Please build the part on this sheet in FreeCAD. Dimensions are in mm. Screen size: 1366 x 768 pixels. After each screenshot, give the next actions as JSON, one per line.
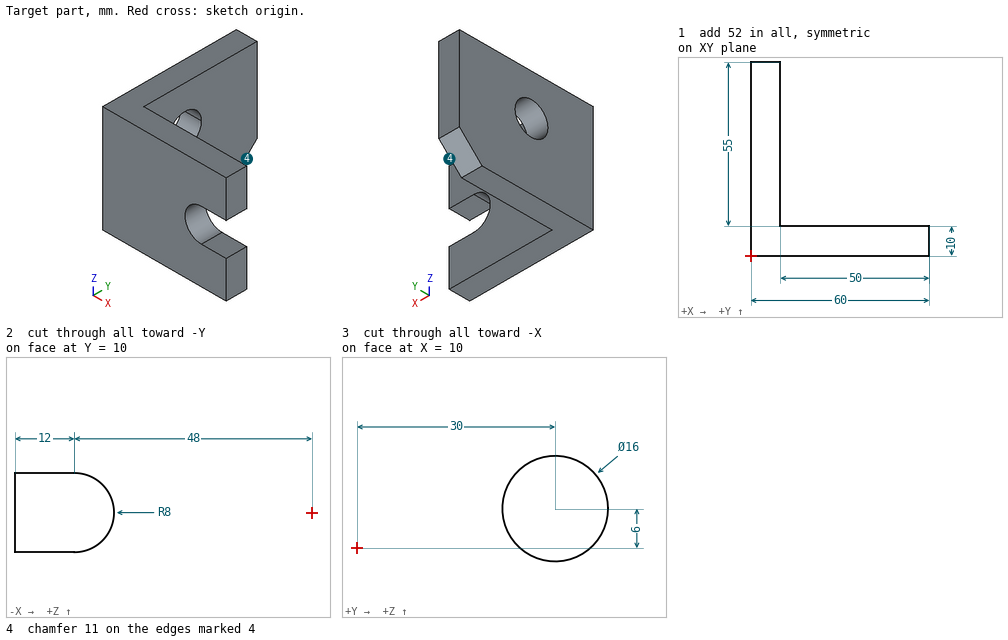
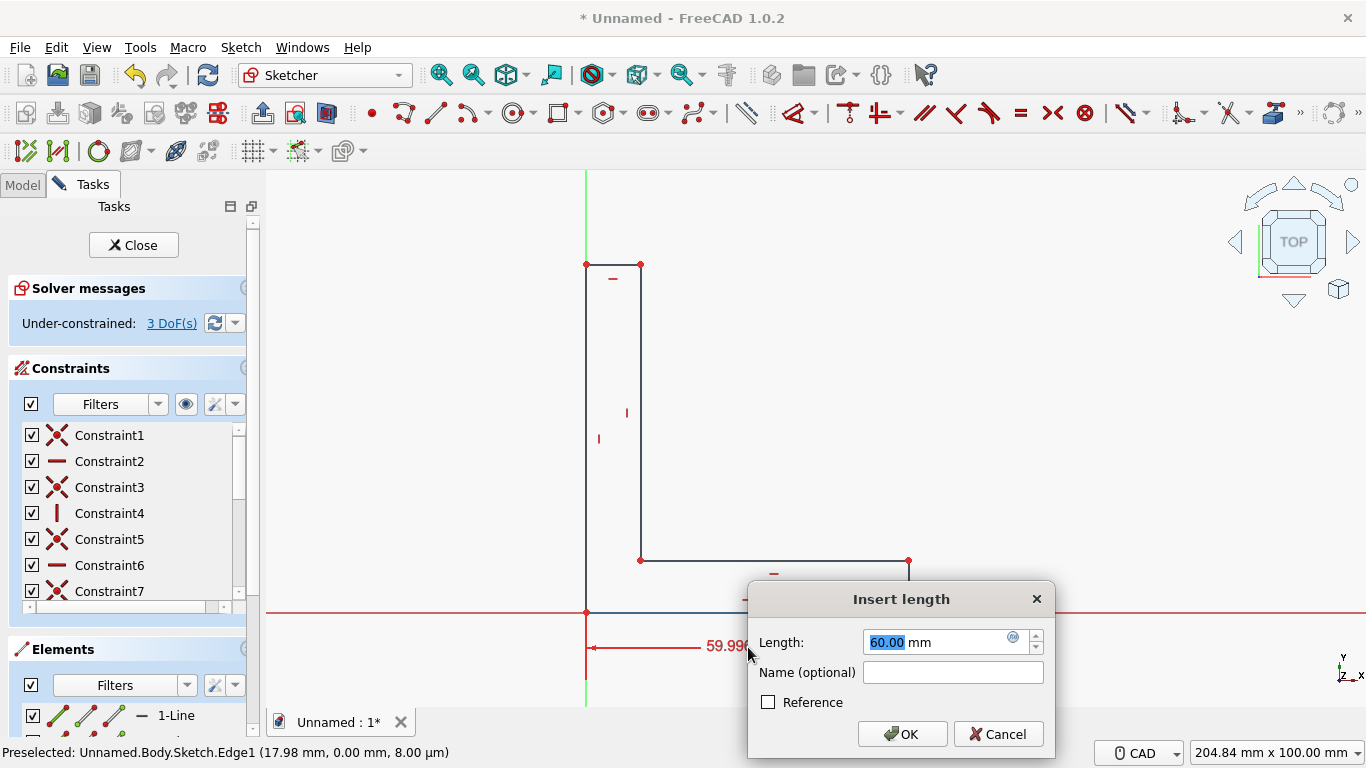
{"action": "type", "text": "60"}
{"action": "key", "text": "Return"}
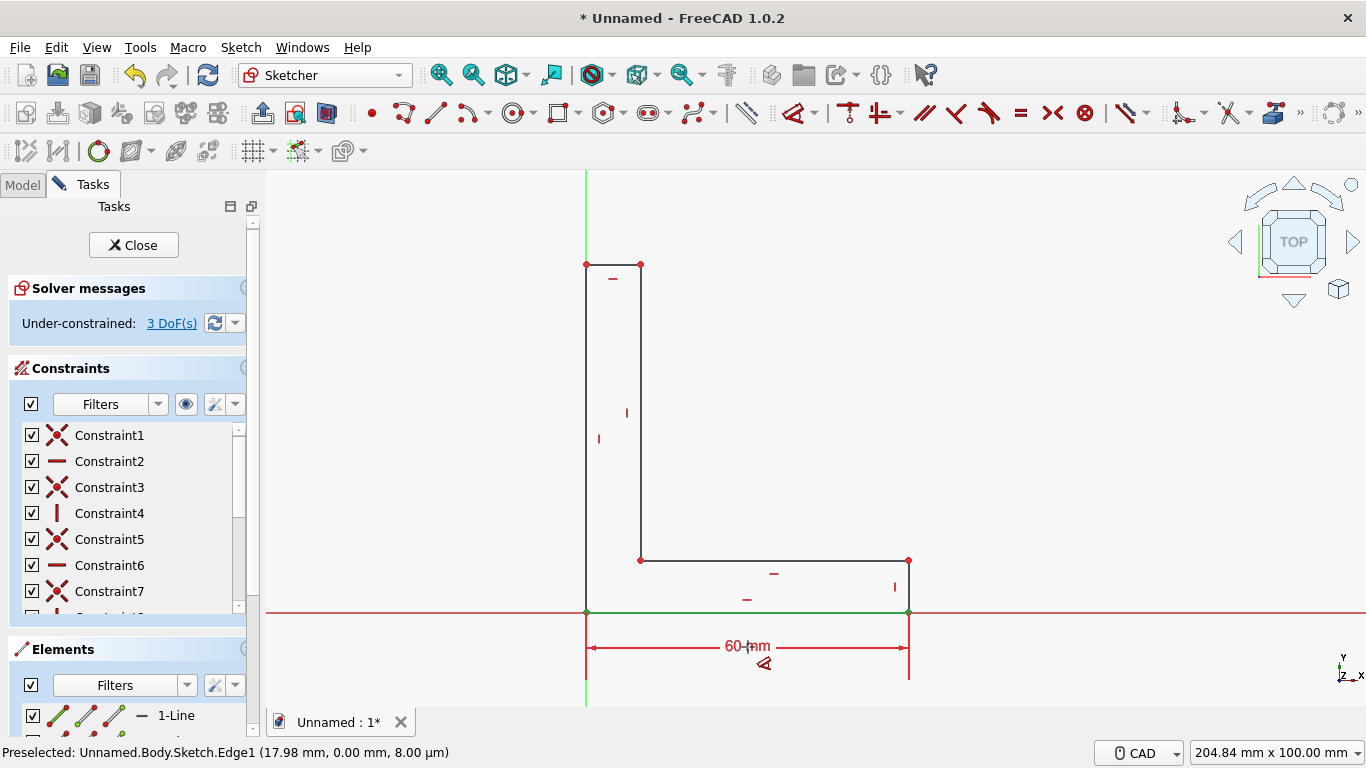
{"action": "left_click", "coordinate": [909, 597]}
{"action": "left_click", "coordinate": [943, 587]}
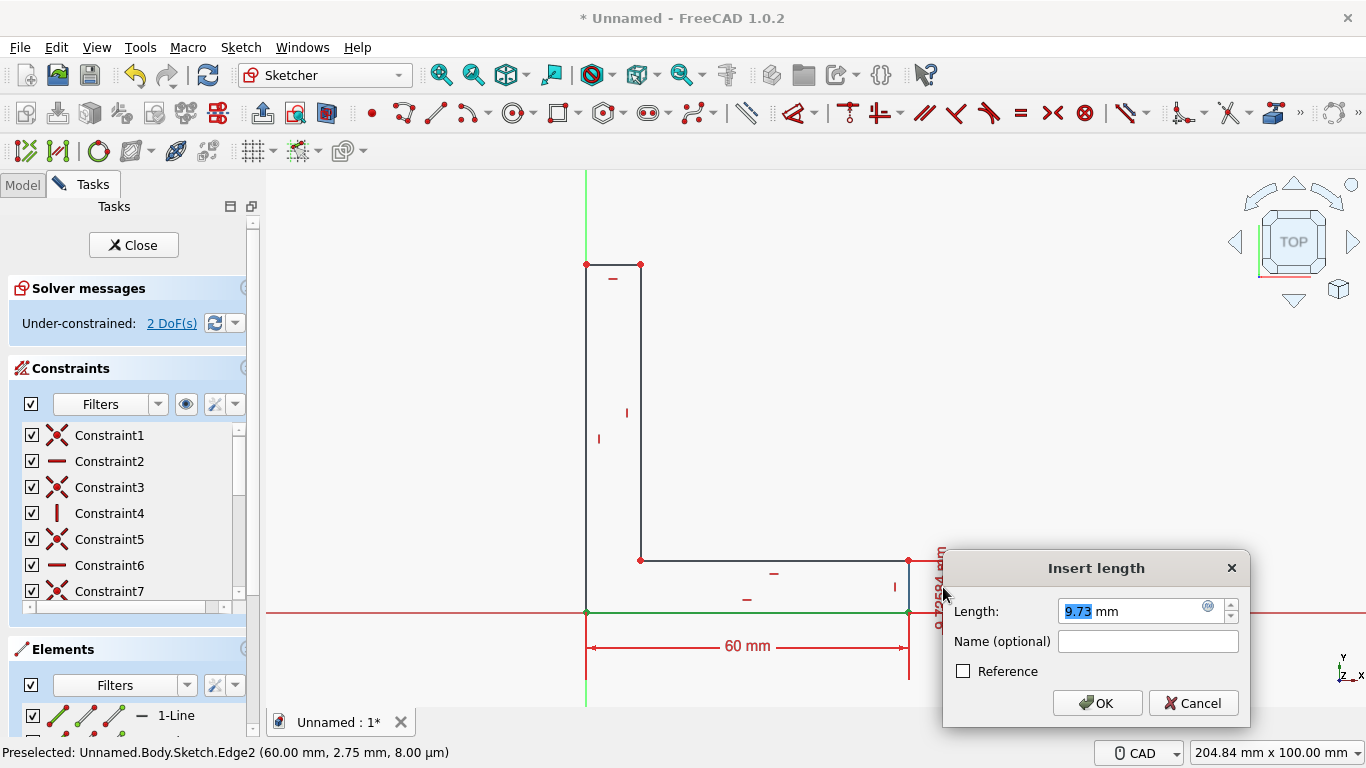
{"action": "type", "text": "10"}
{"action": "key", "text": "Return"}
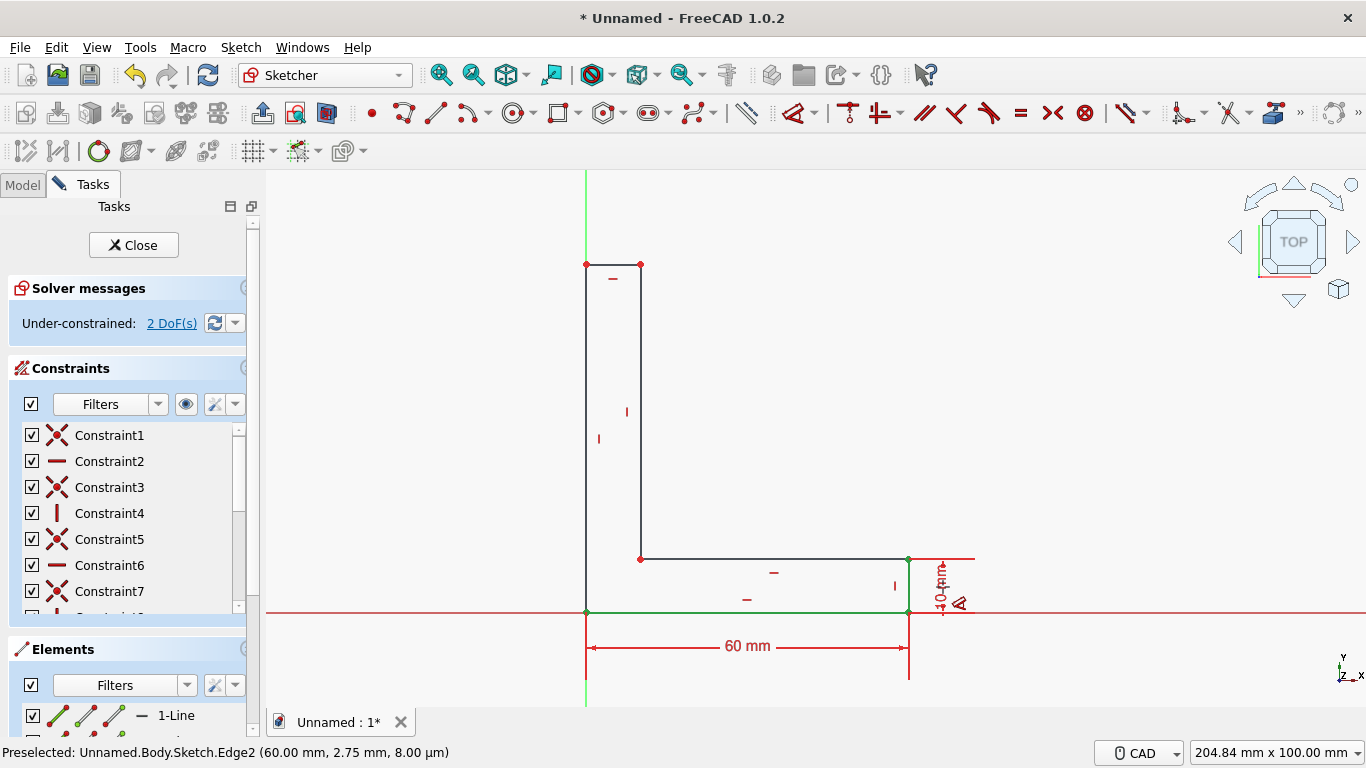
{"action": "left_click", "coordinate": [828, 559]}
{"action": "left_click", "coordinate": [775, 593]}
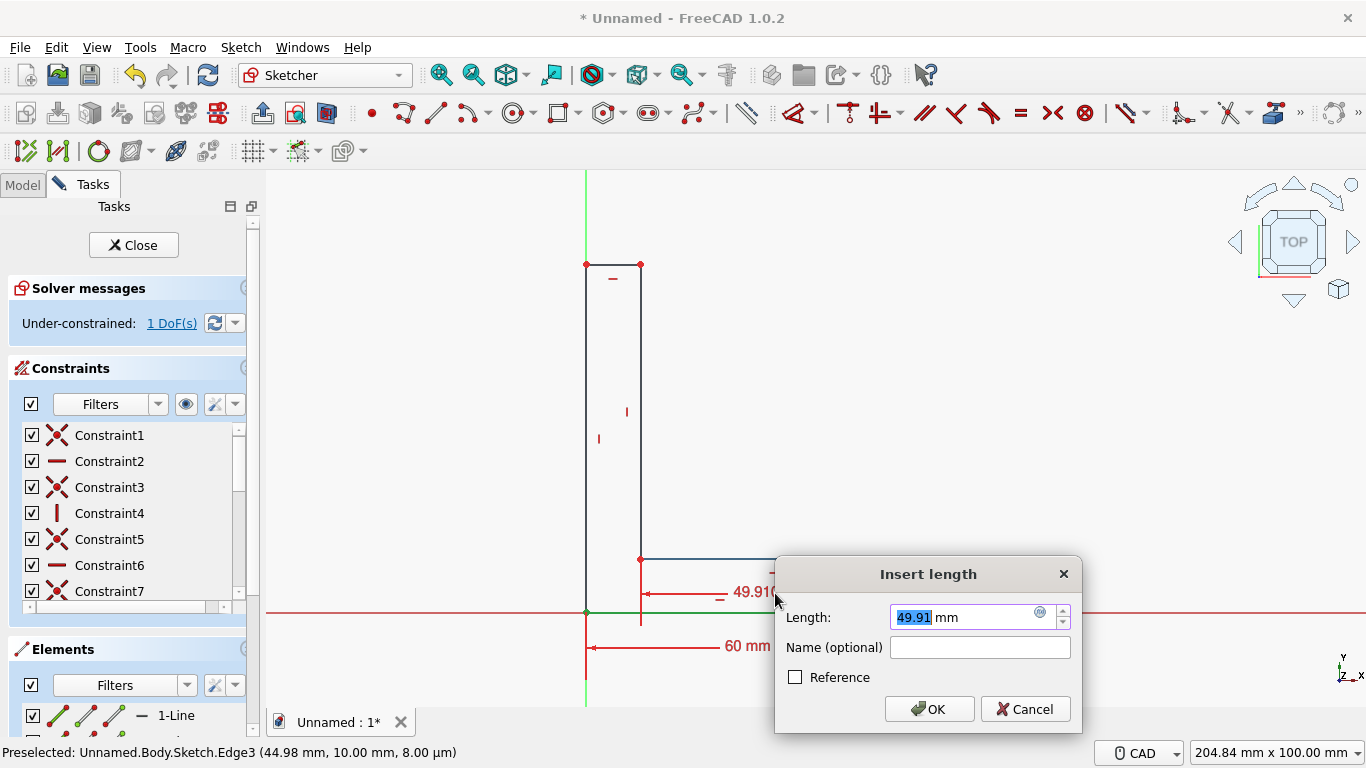
{"action": "type", "text": "50"}
{"action": "key", "text": "Return"}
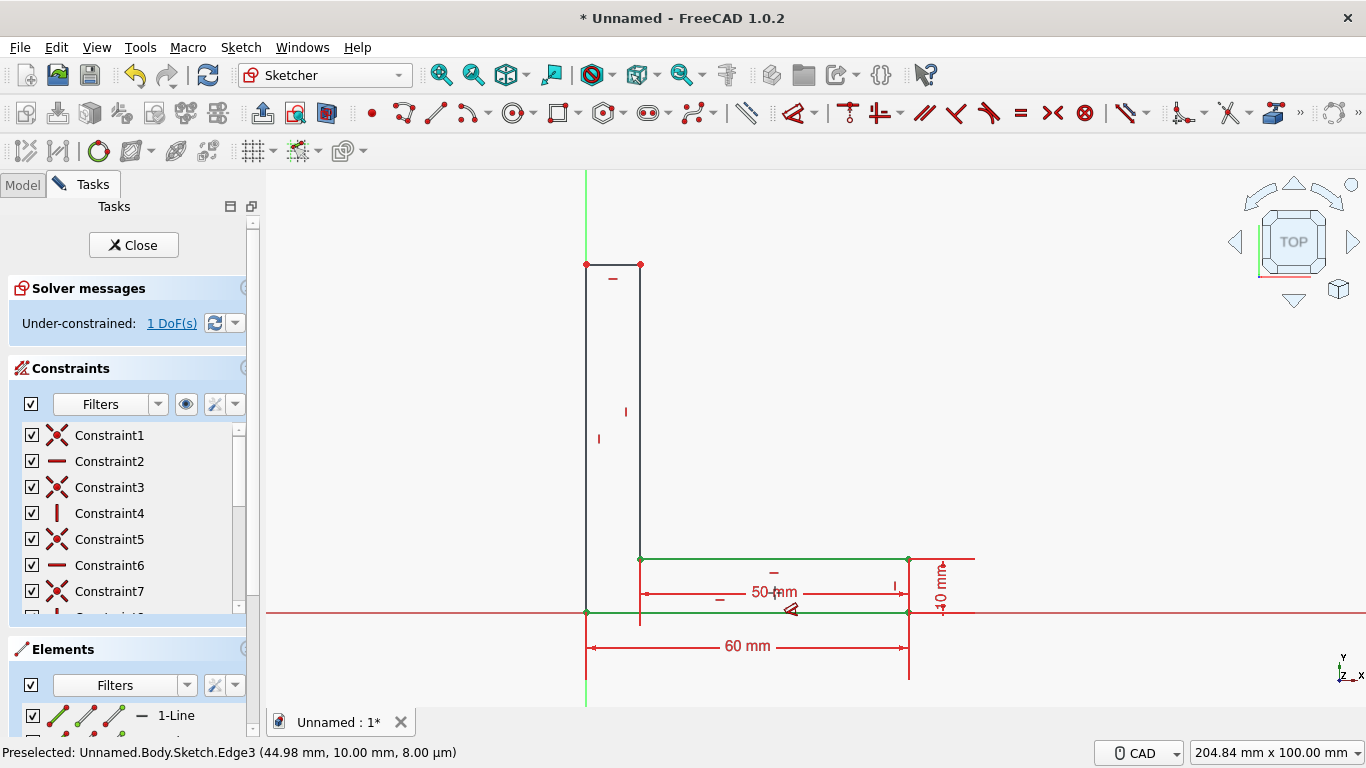
{"action": "left_click", "coordinate": [640, 471]}
{"action": "left_click", "coordinate": [606, 412]}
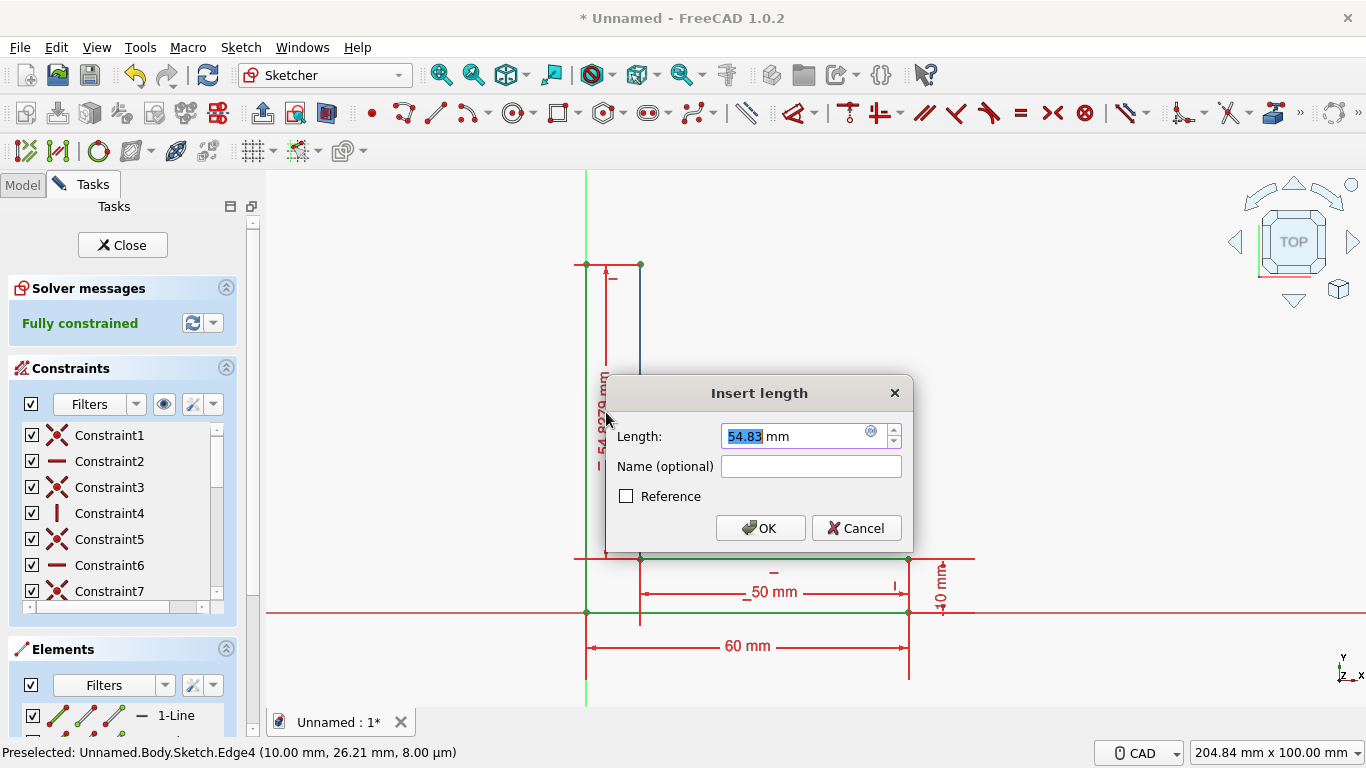
{"action": "type", "text": "55"}
{"action": "key", "text": "Return"}
{"action": "key", "text": "Escape"}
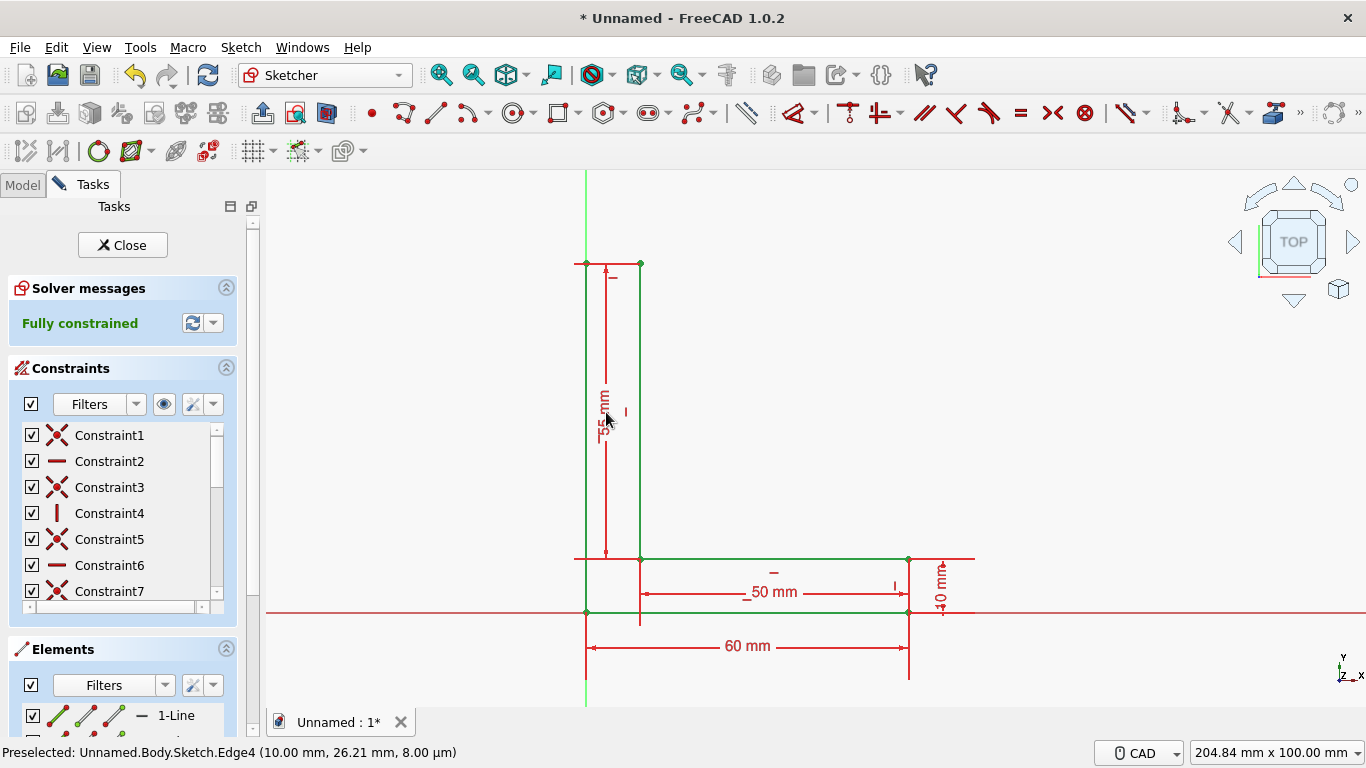
{"action": "left_click", "coordinate": [123, 245]}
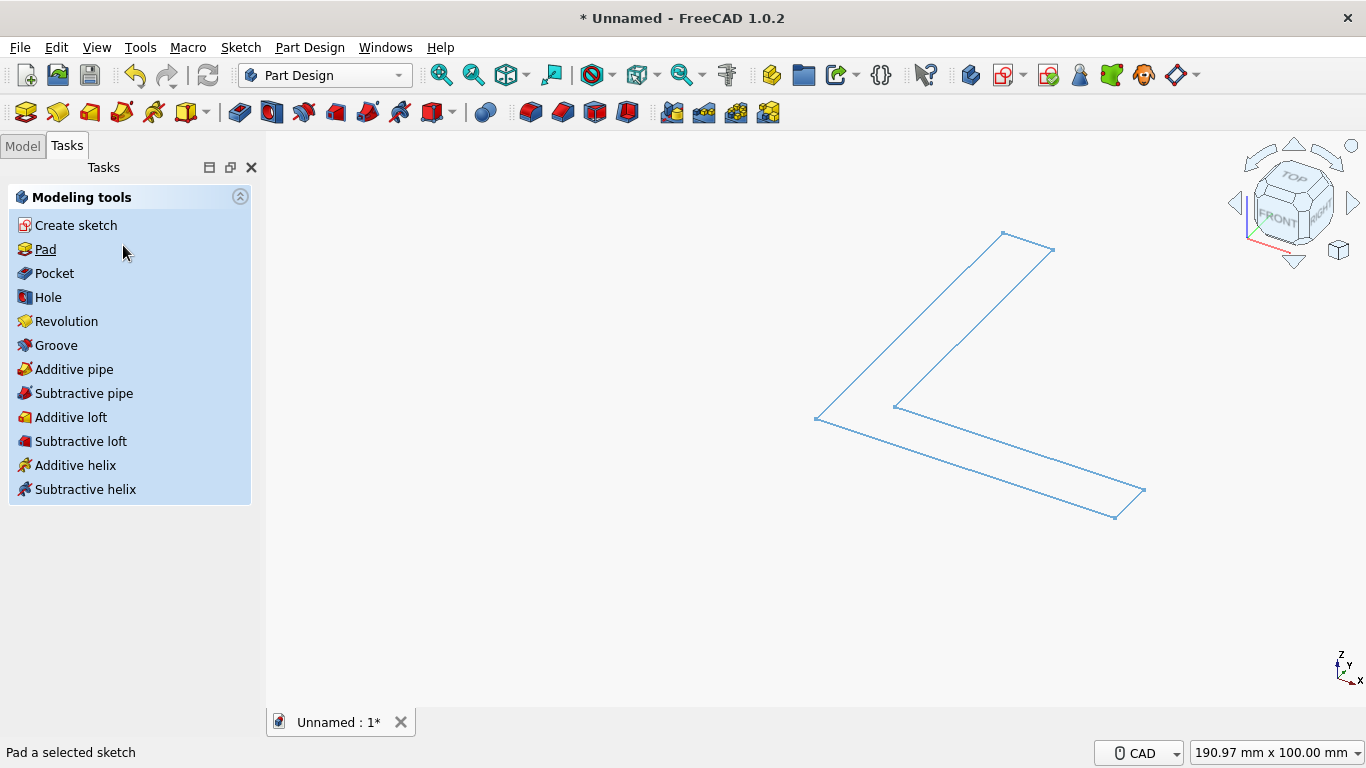
{"action": "left_click", "coordinate": [26, 112]}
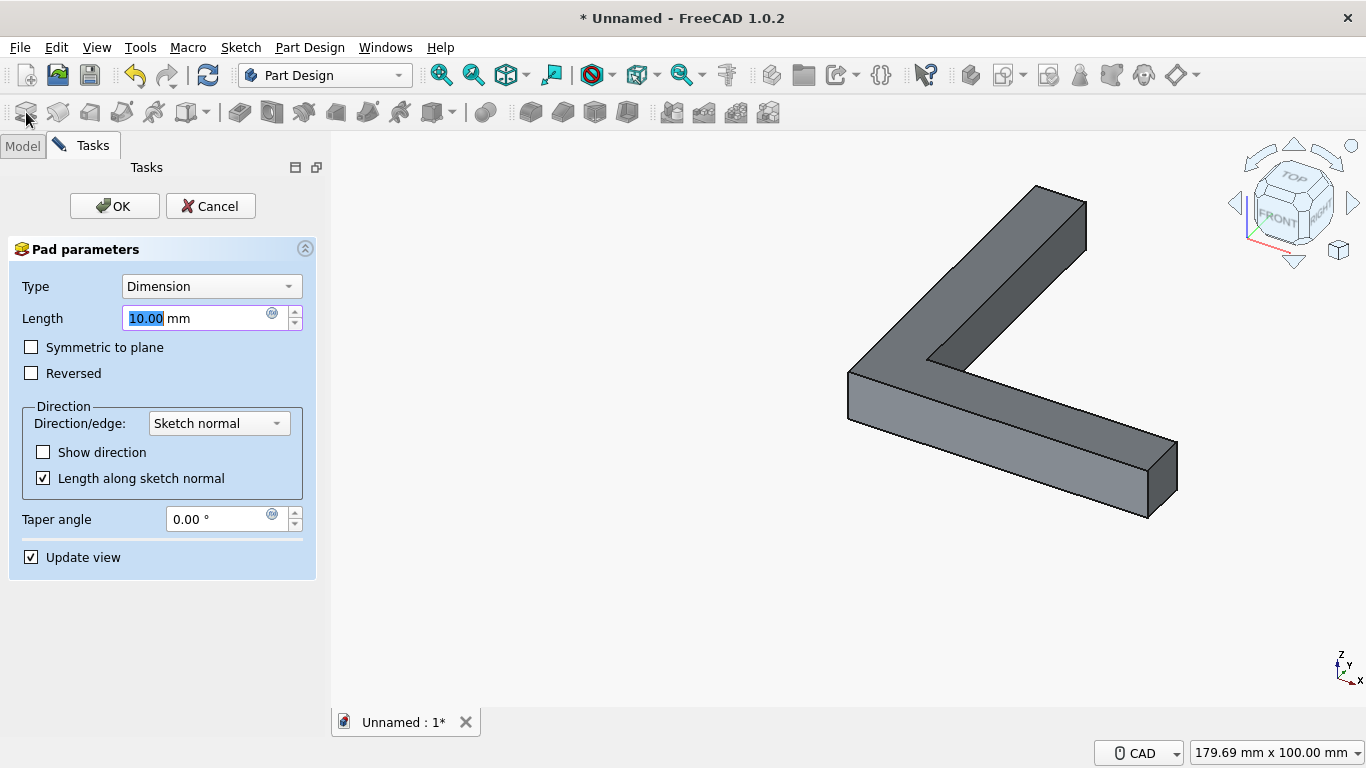
{"action": "type", "text": "52"}
{"action": "key", "text": "Tab"}